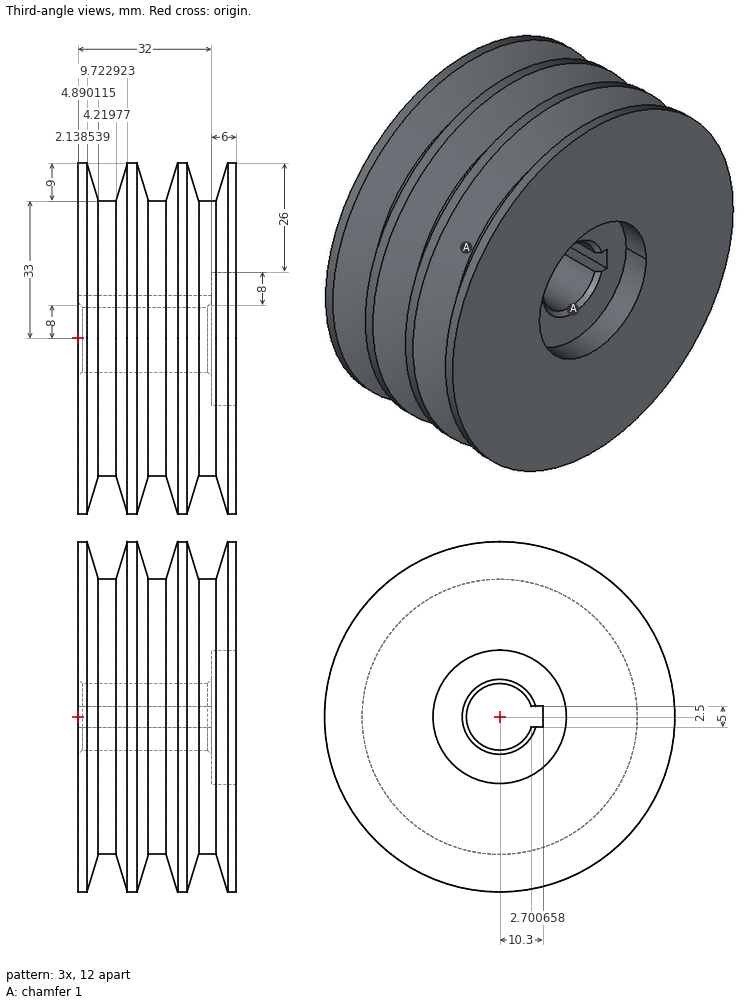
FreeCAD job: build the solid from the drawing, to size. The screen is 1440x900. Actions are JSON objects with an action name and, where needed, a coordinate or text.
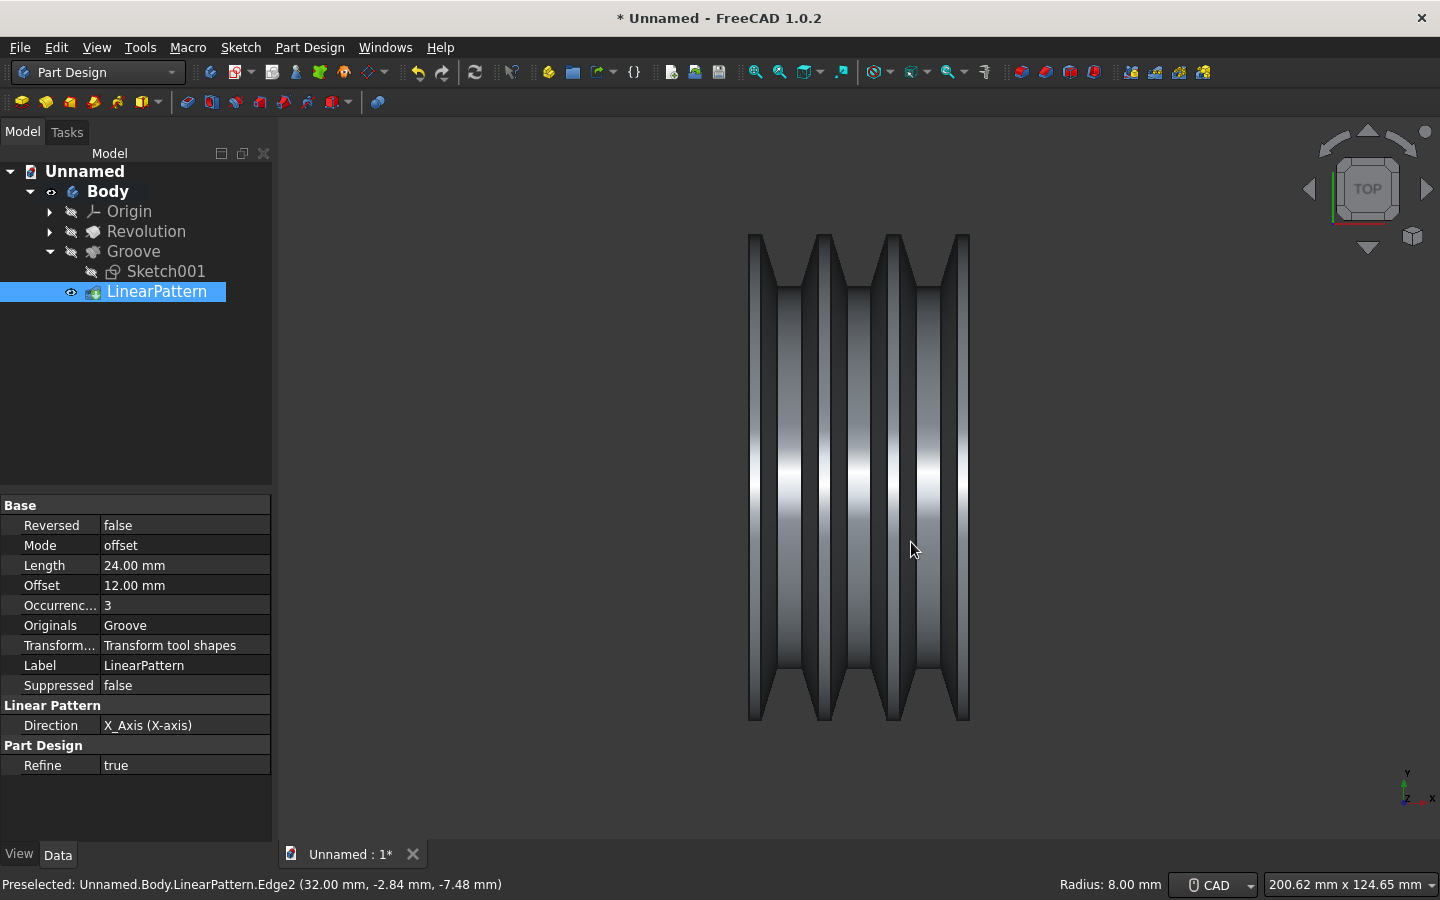
{"action": "key", "text": "1"}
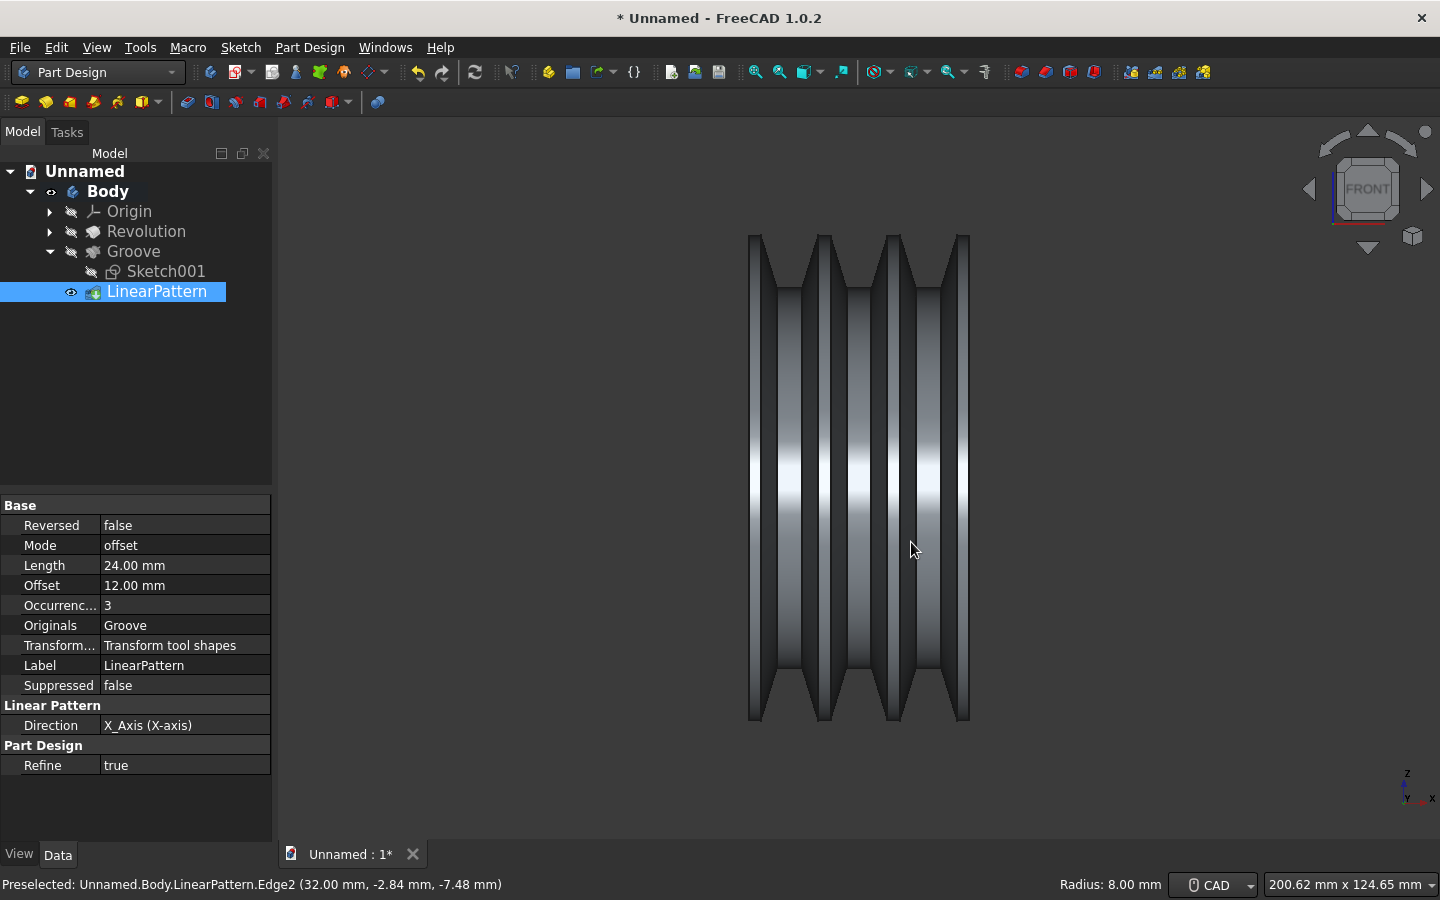
{"action": "key", "text": "3"}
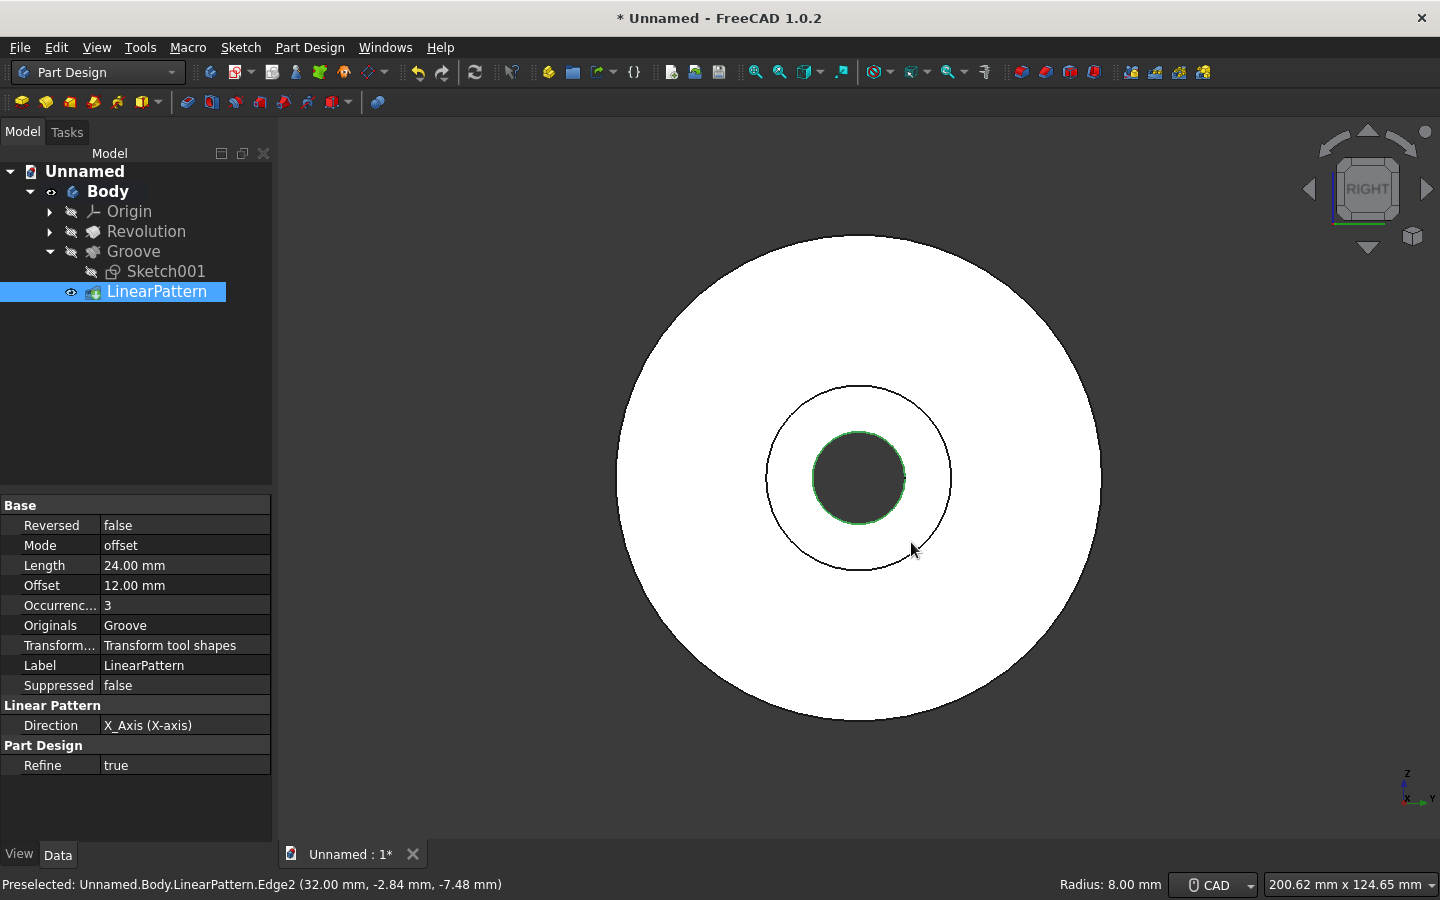
{"action": "key", "text": "5"}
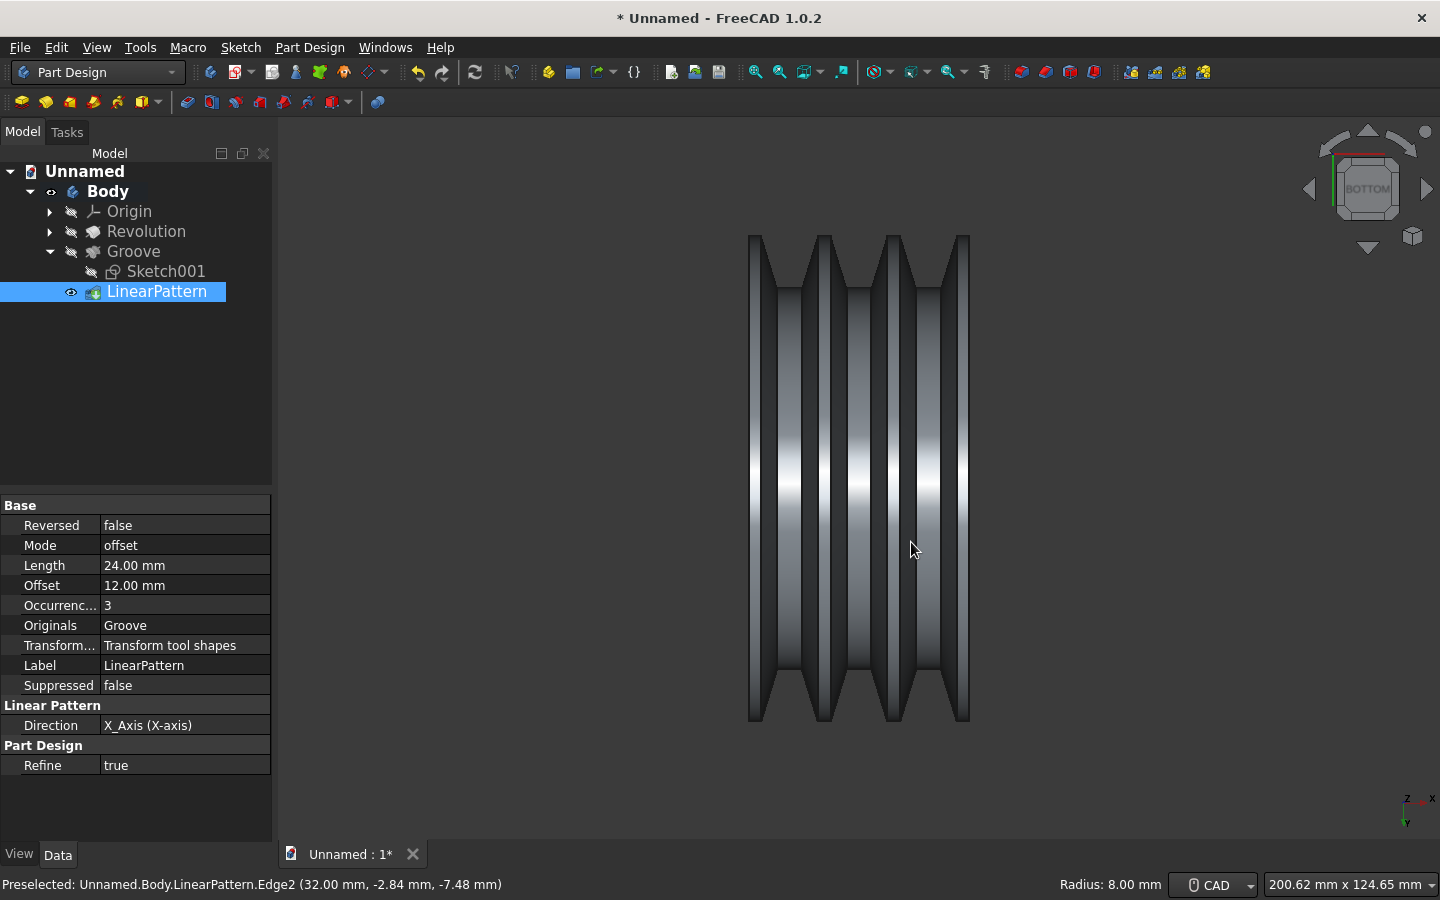
{"action": "key", "text": "4"}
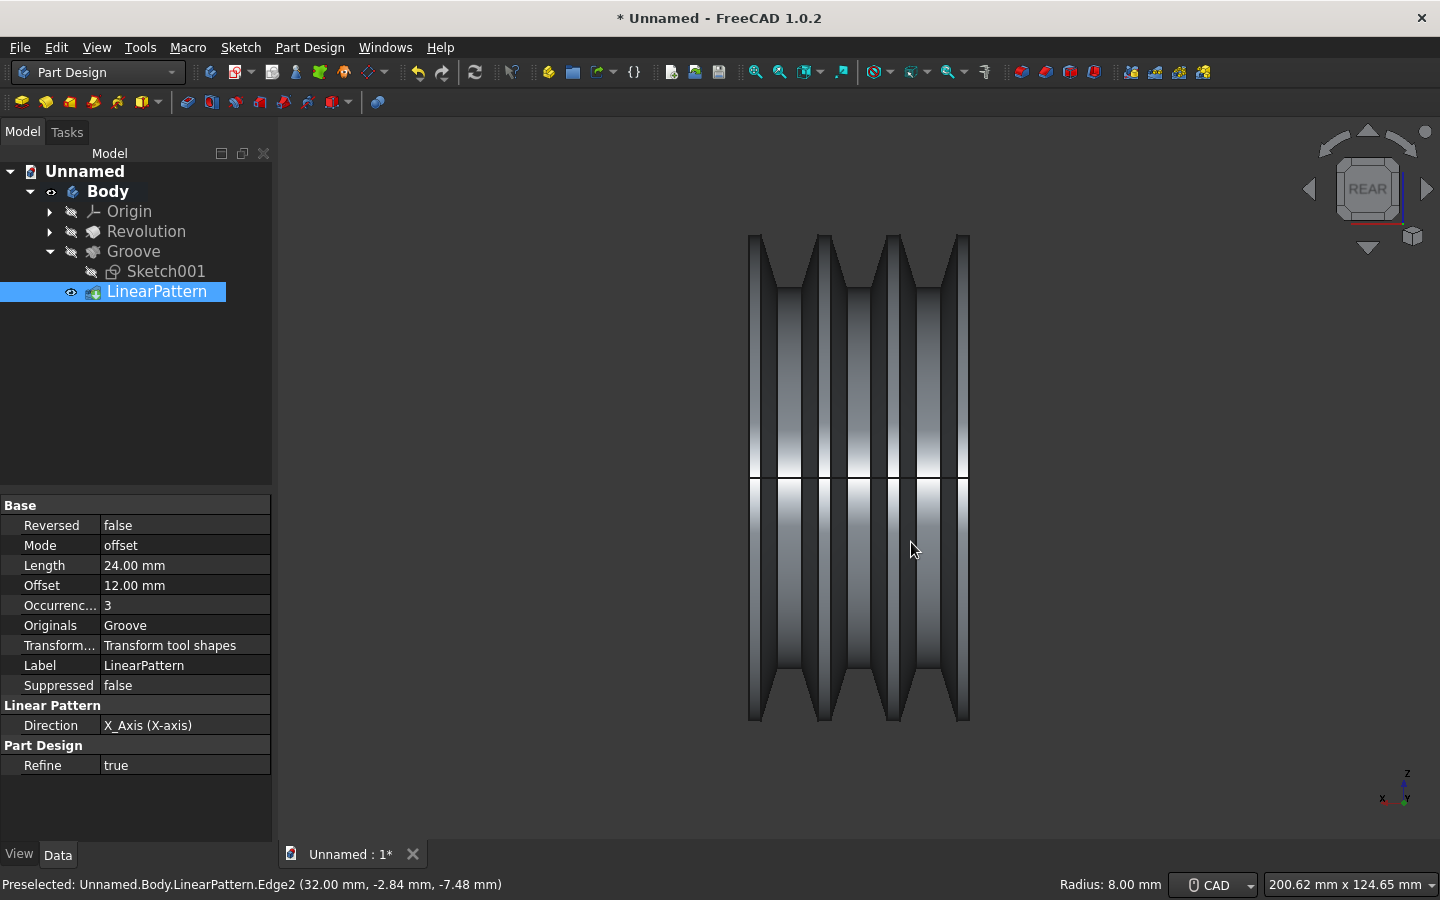
{"action": "key", "text": "6"}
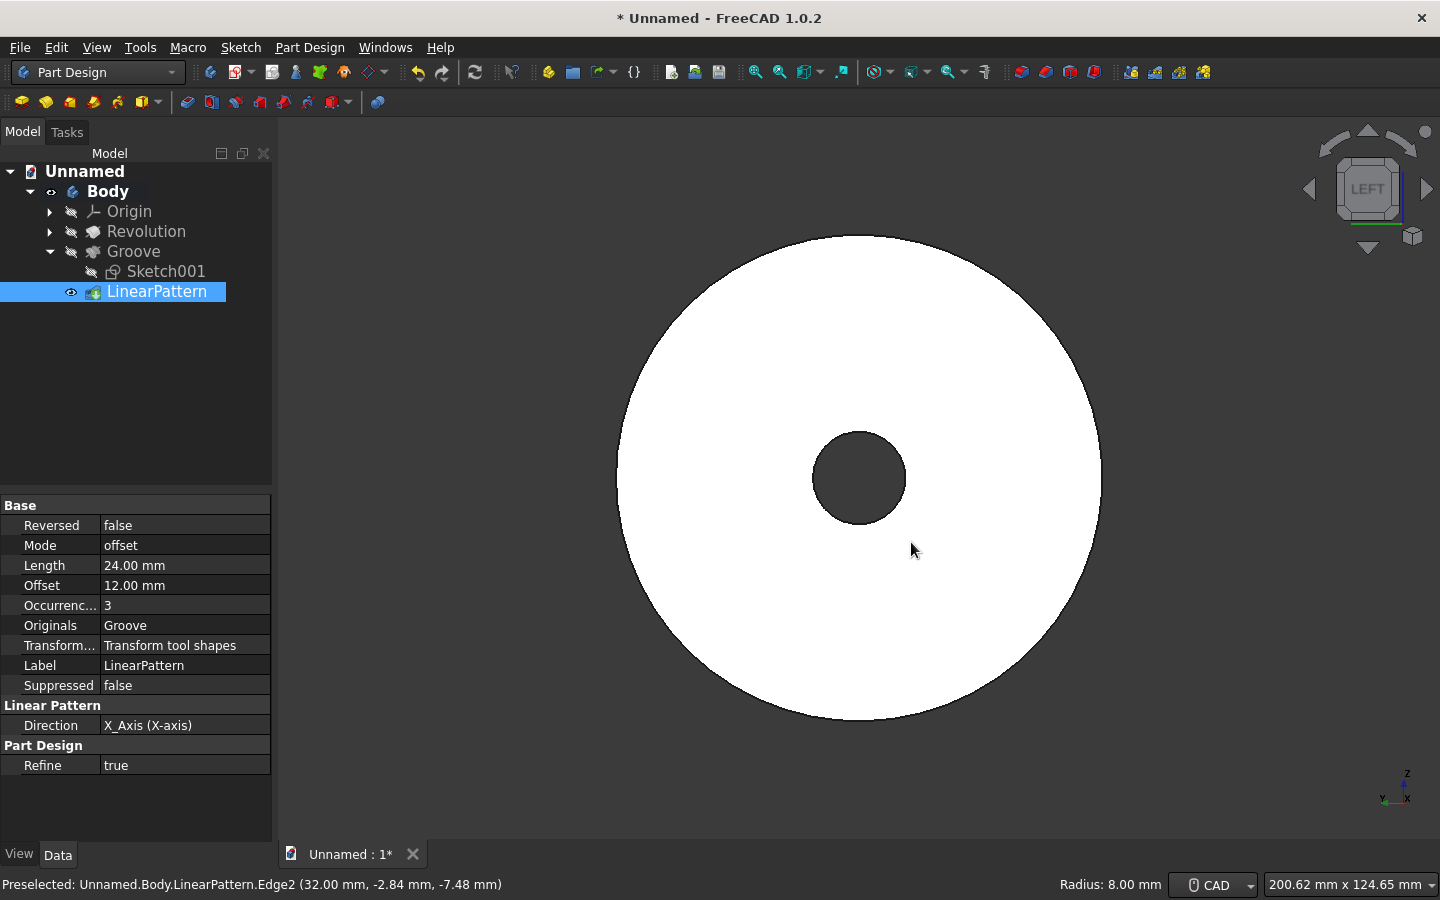
{"action": "left_click", "coordinate": [897, 450], "text": "ctrl"}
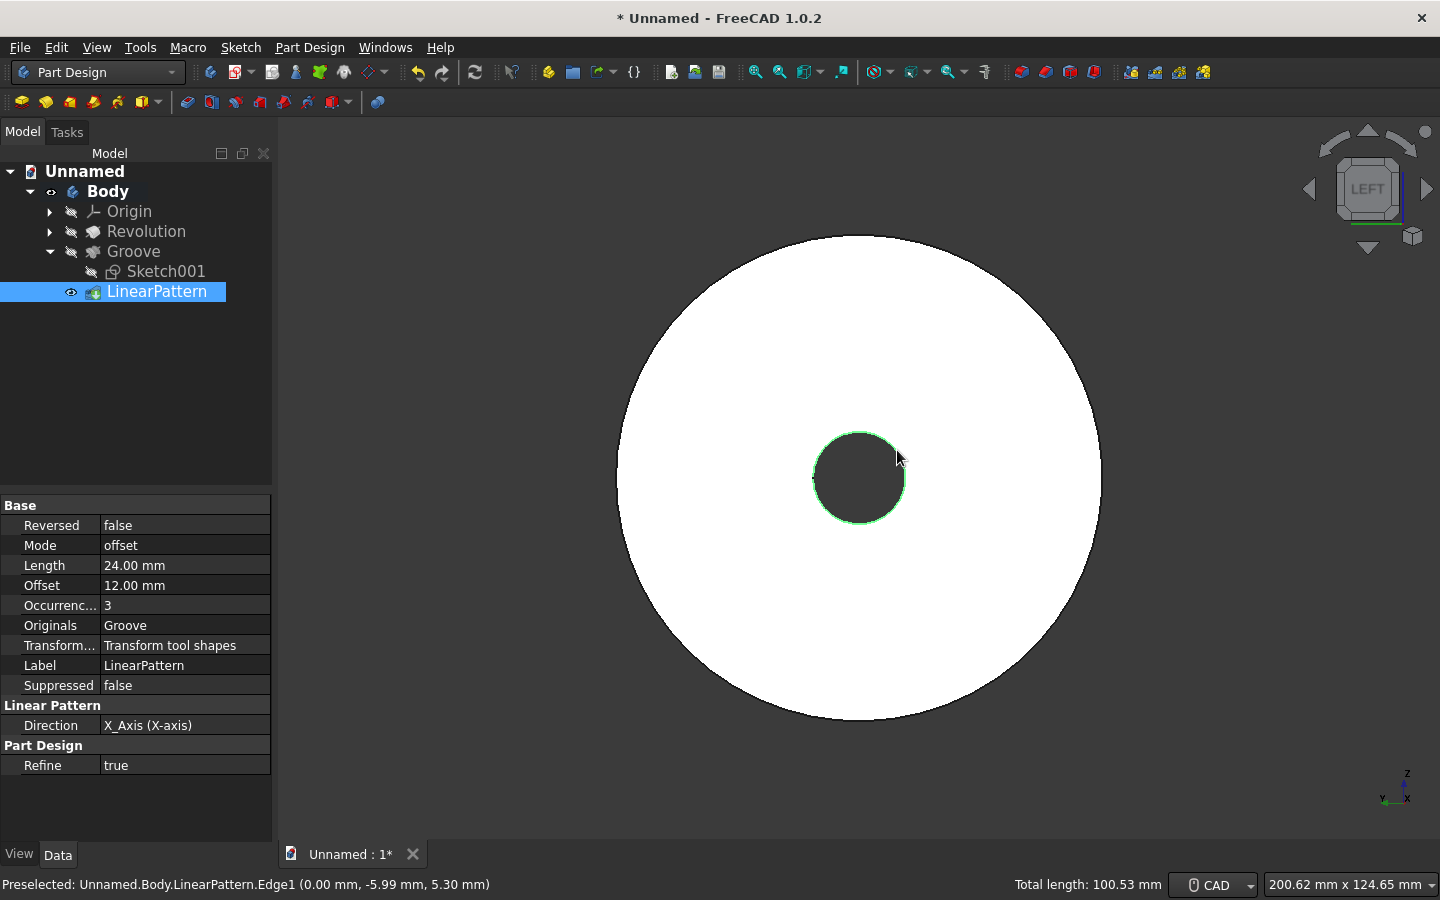
{"action": "left_click", "coordinate": [1046, 72]}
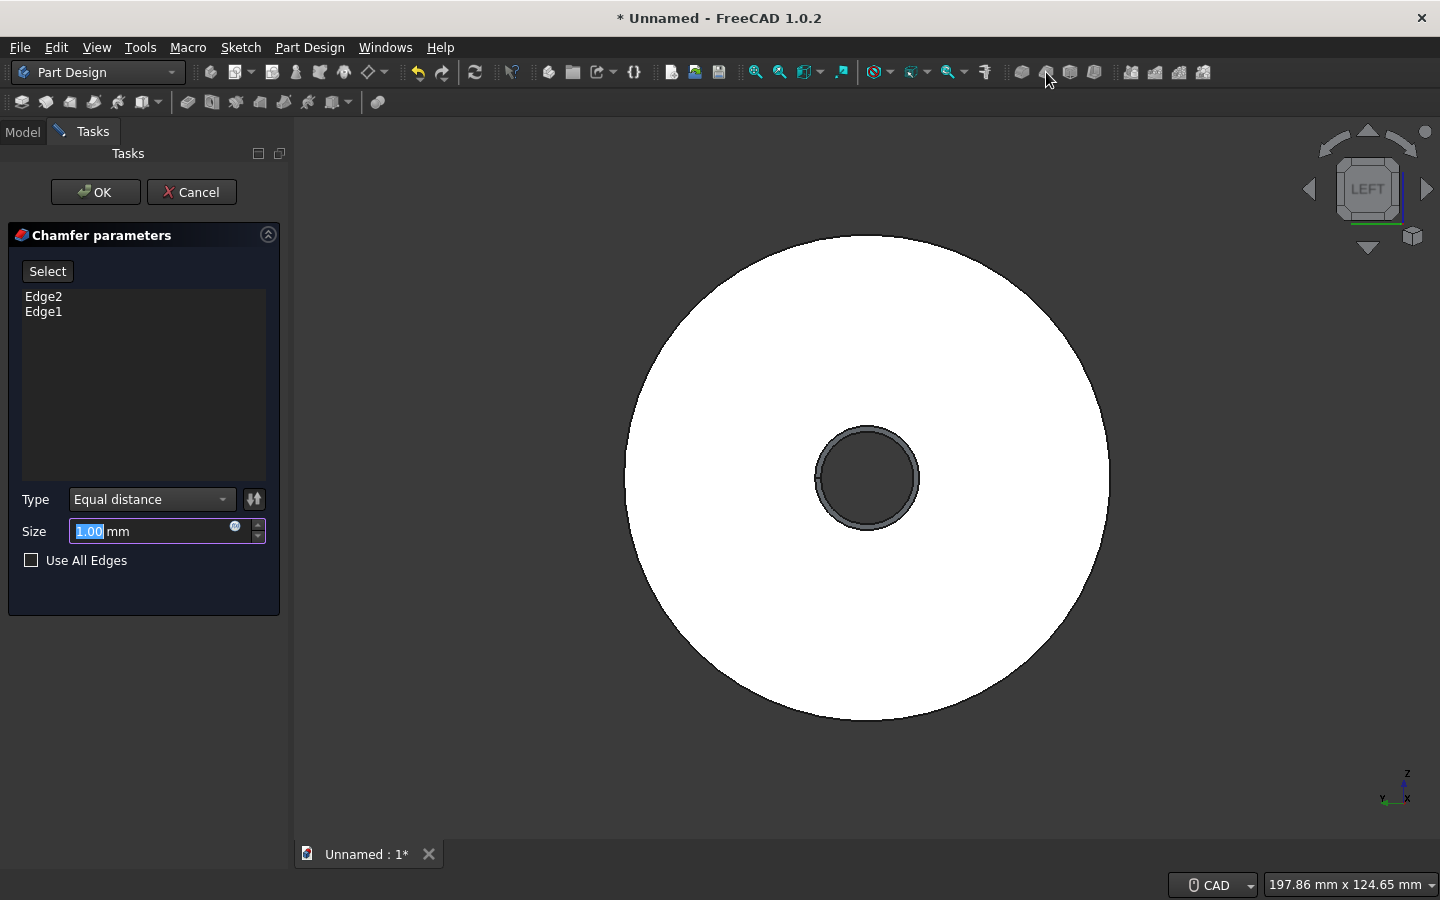
{"action": "type", "text": "1"}
{"action": "key", "text": "Tab"}